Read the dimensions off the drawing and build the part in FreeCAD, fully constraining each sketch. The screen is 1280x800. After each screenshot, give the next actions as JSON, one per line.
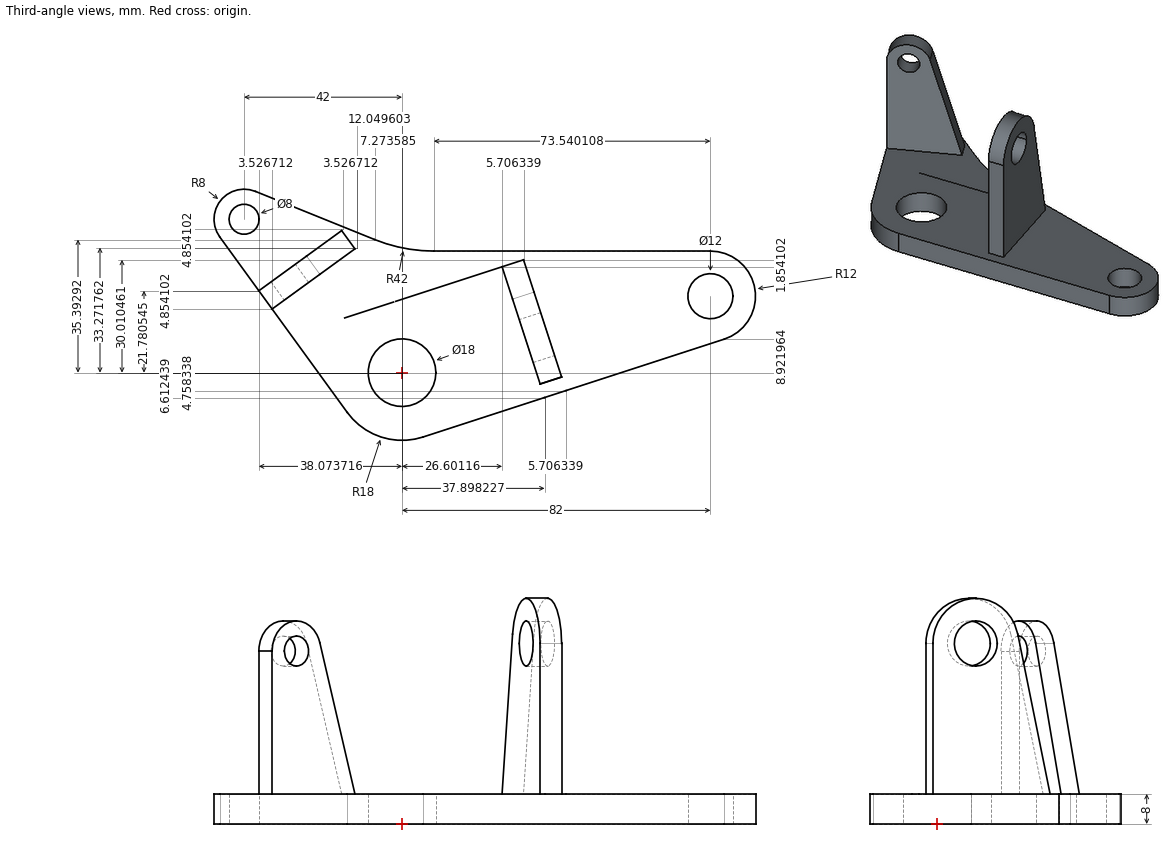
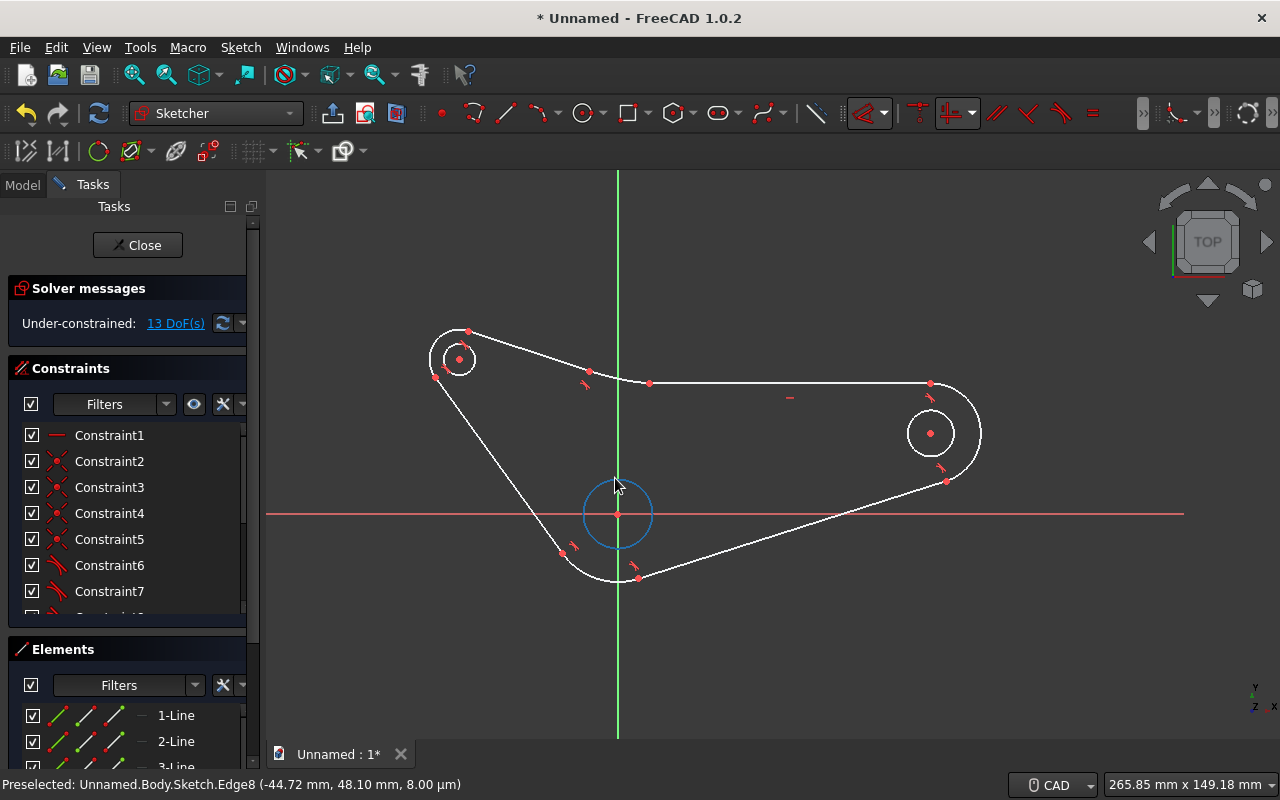
{"action": "left_click", "coordinate": [581, 571]}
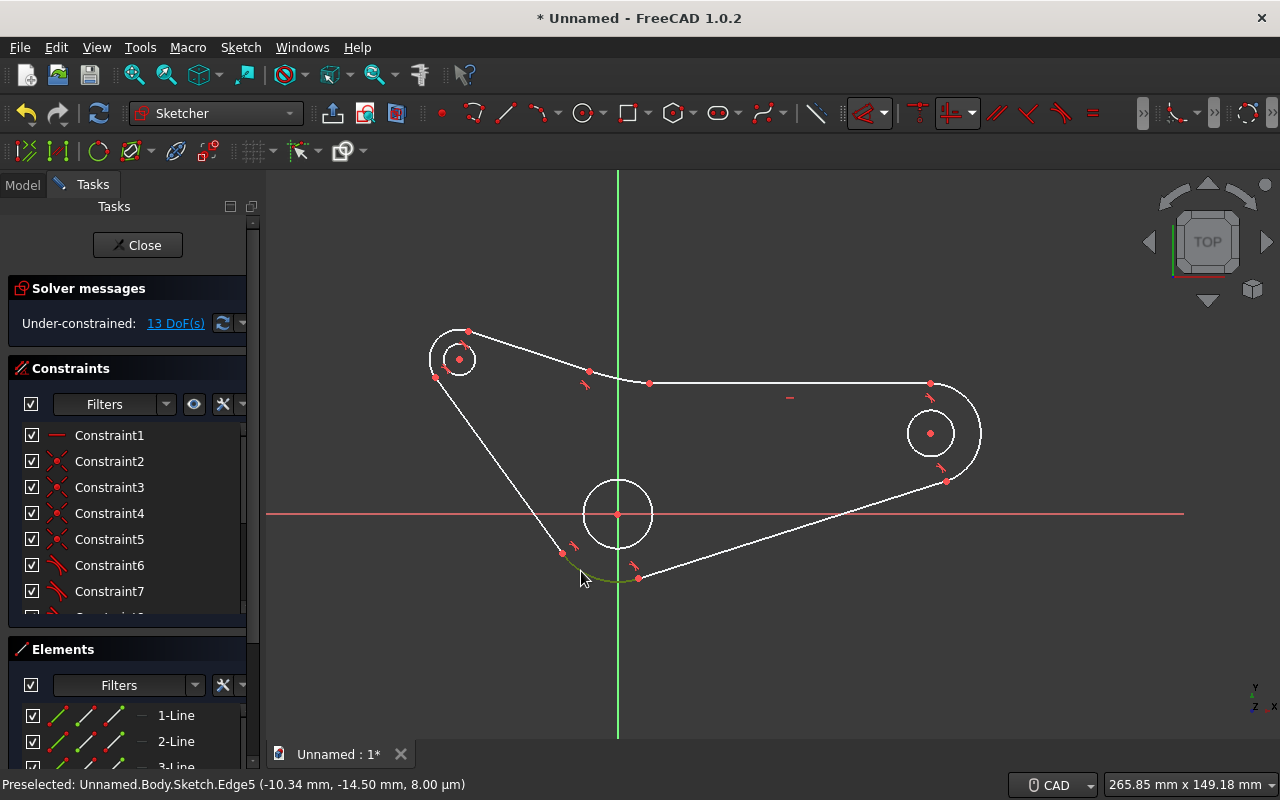
{"action": "key", "text": "k r"}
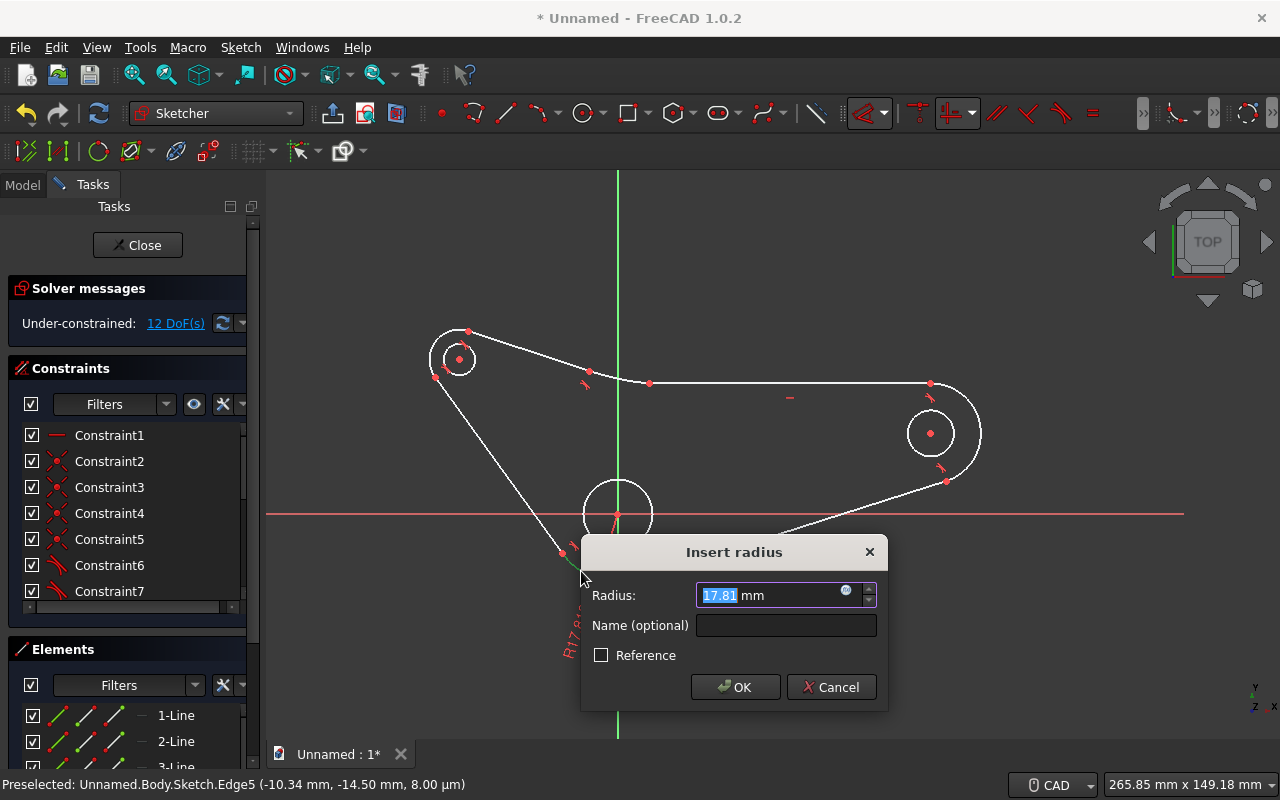
{"action": "type", "text": "18"}
{"action": "key", "text": "Return"}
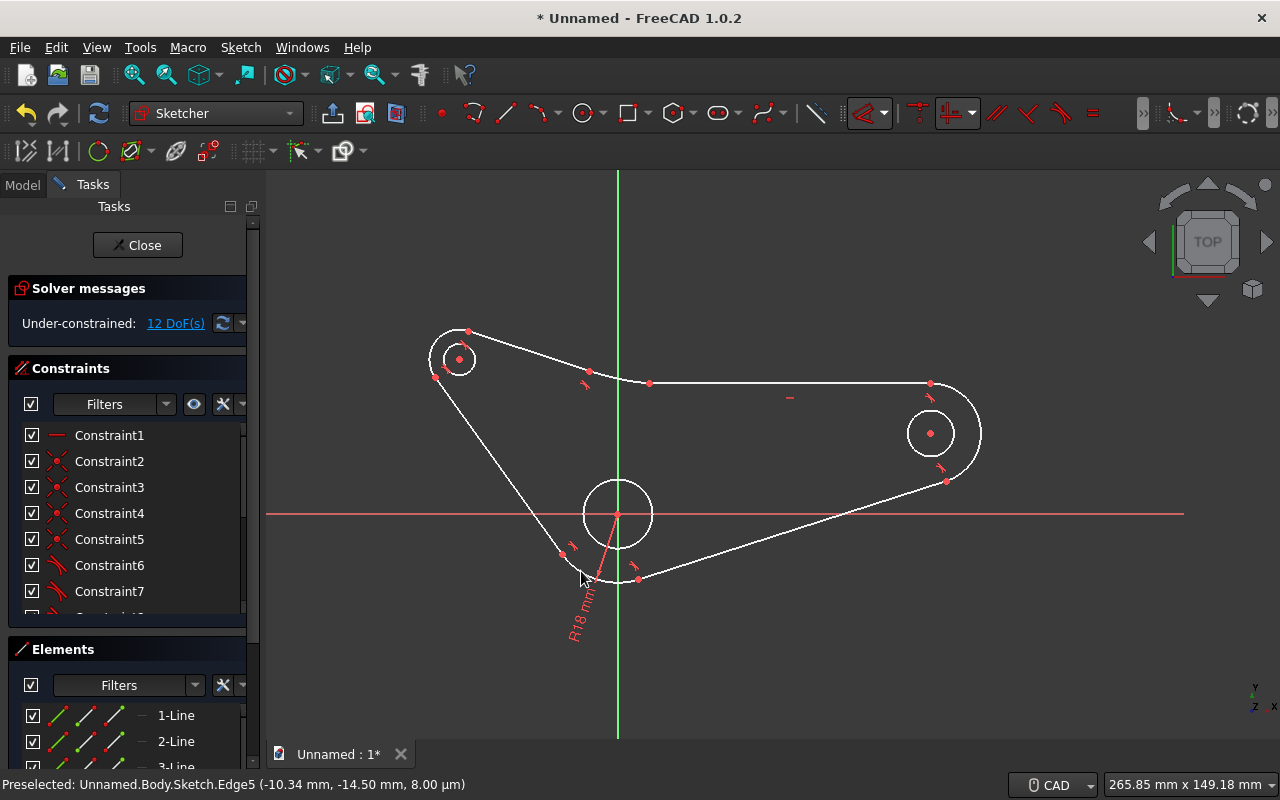
{"action": "left_click", "coordinate": [977, 453]}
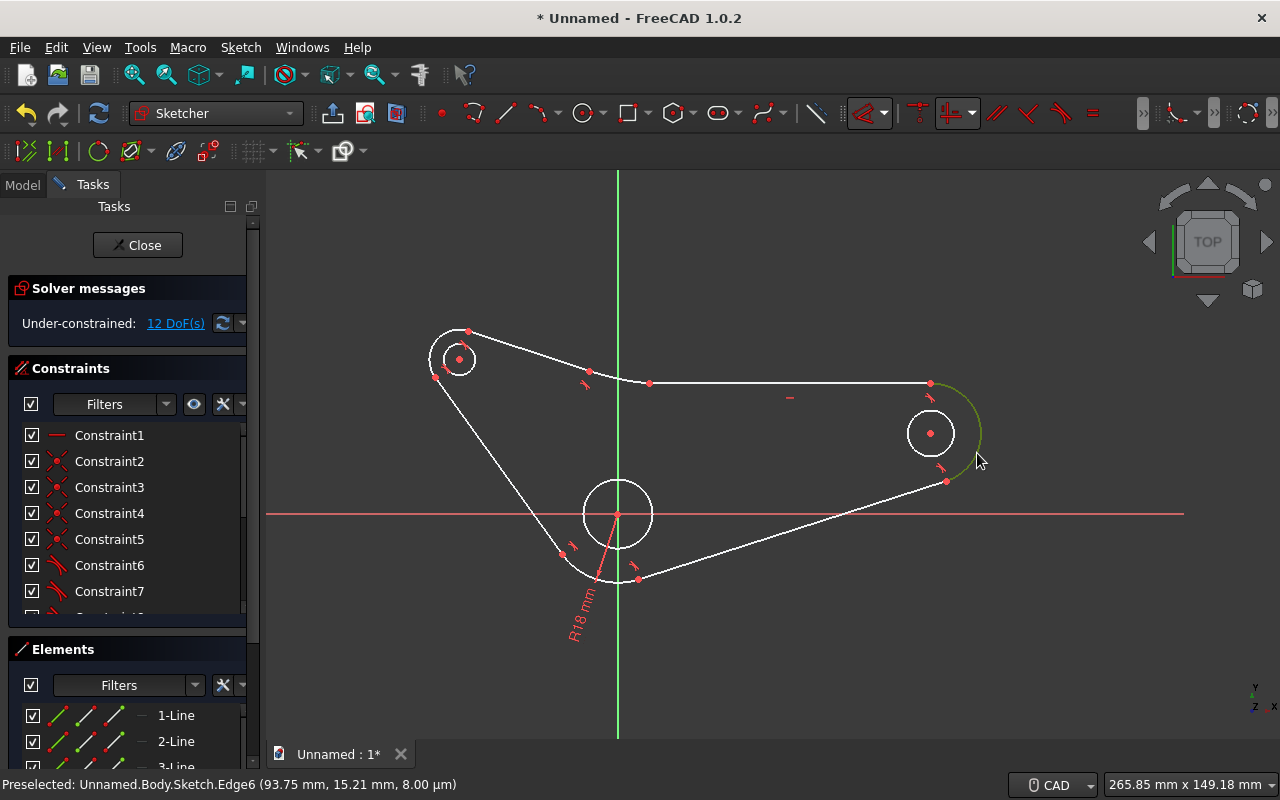
{"action": "left_click", "coordinate": [886, 114]}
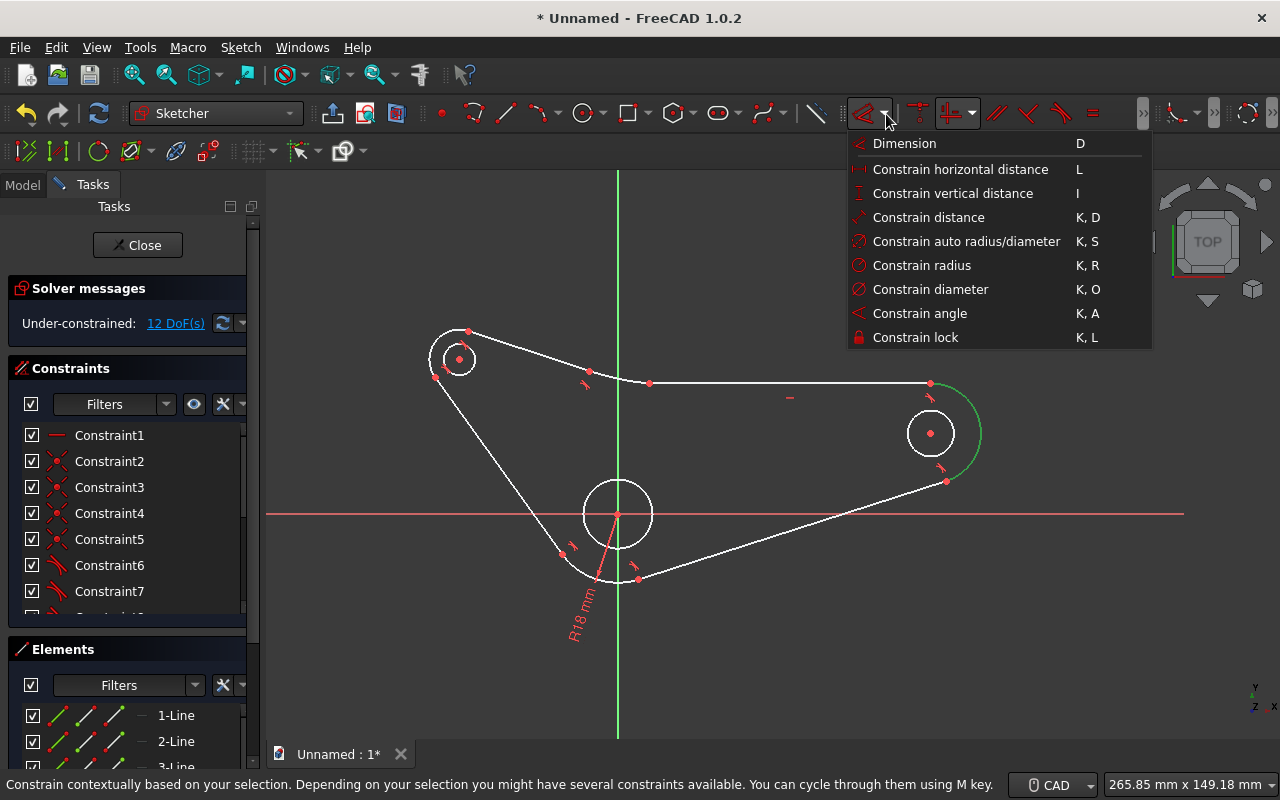
{"action": "left_click", "coordinate": [1000, 265]}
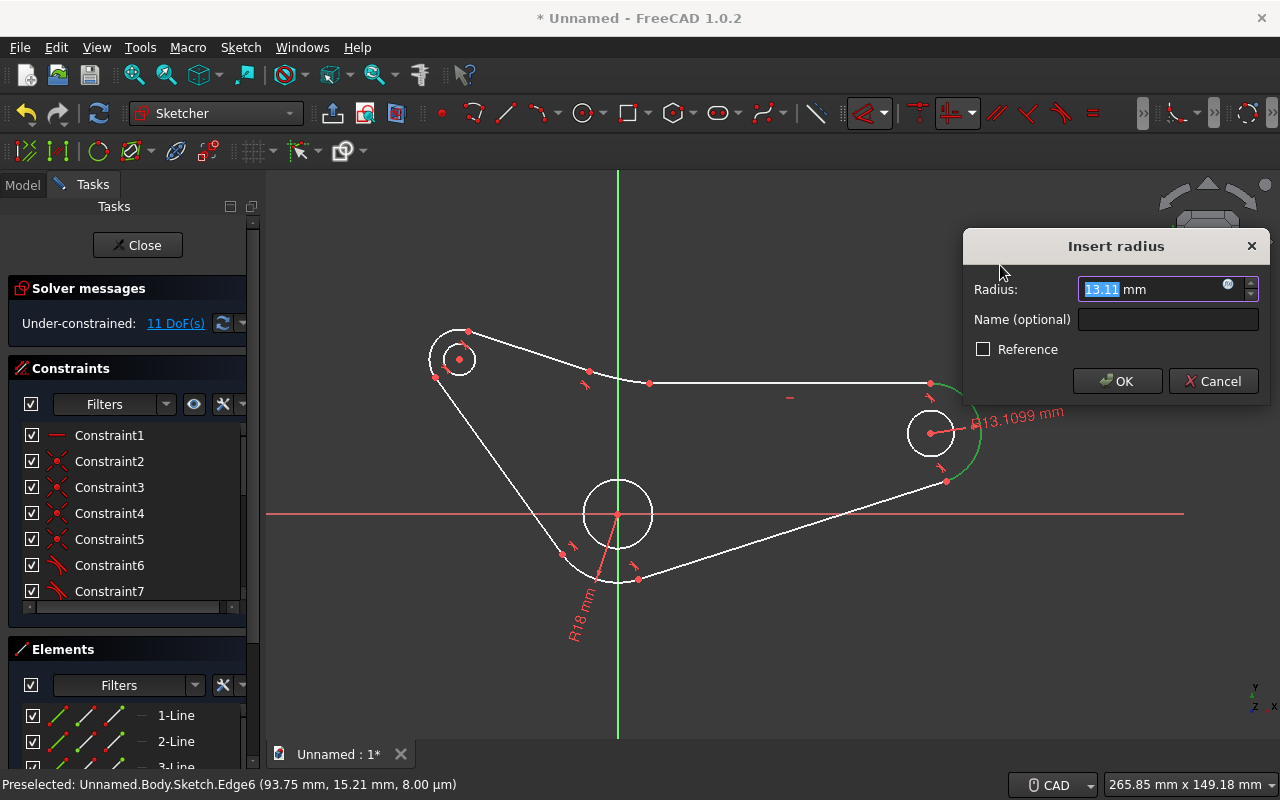
{"action": "type", "text": "12"}
{"action": "key", "text": "Return"}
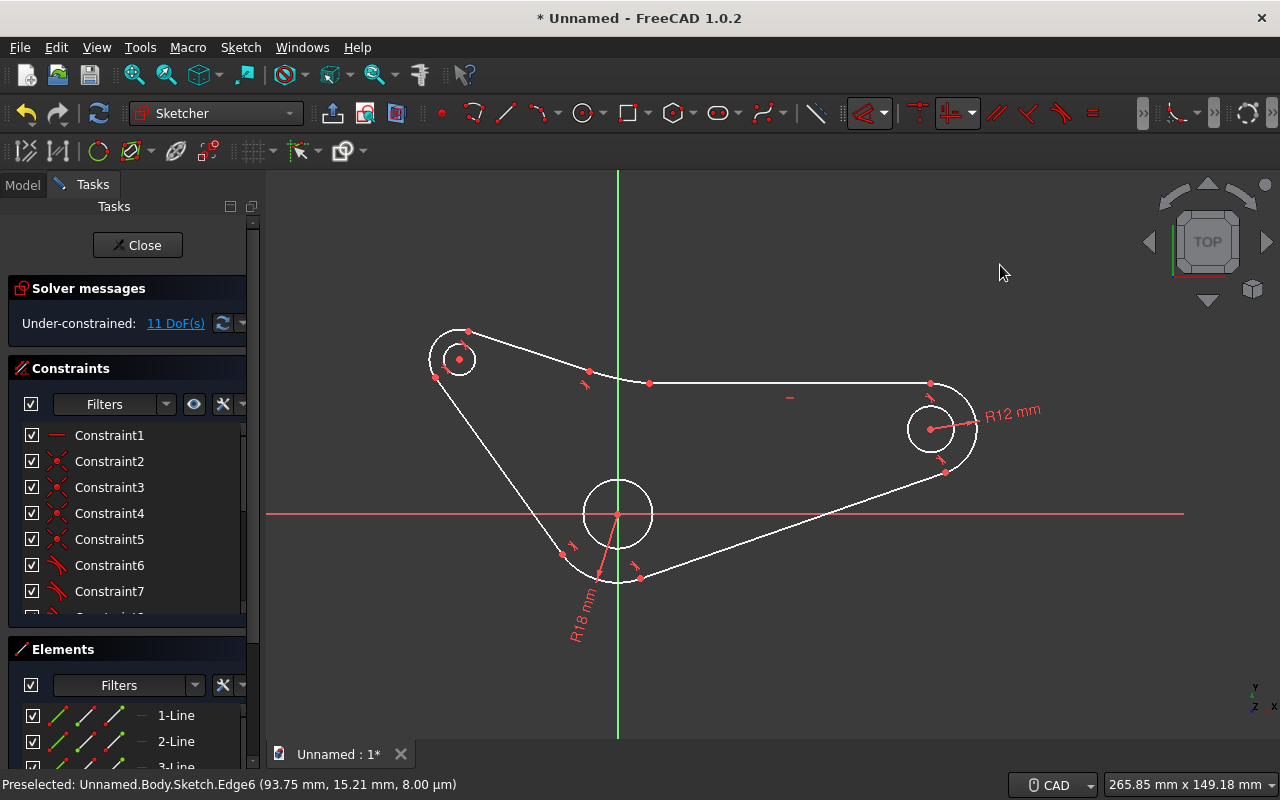
{"action": "scroll", "coordinate": [608, 376], "scroll_direction": "up", "scroll_amount": 2}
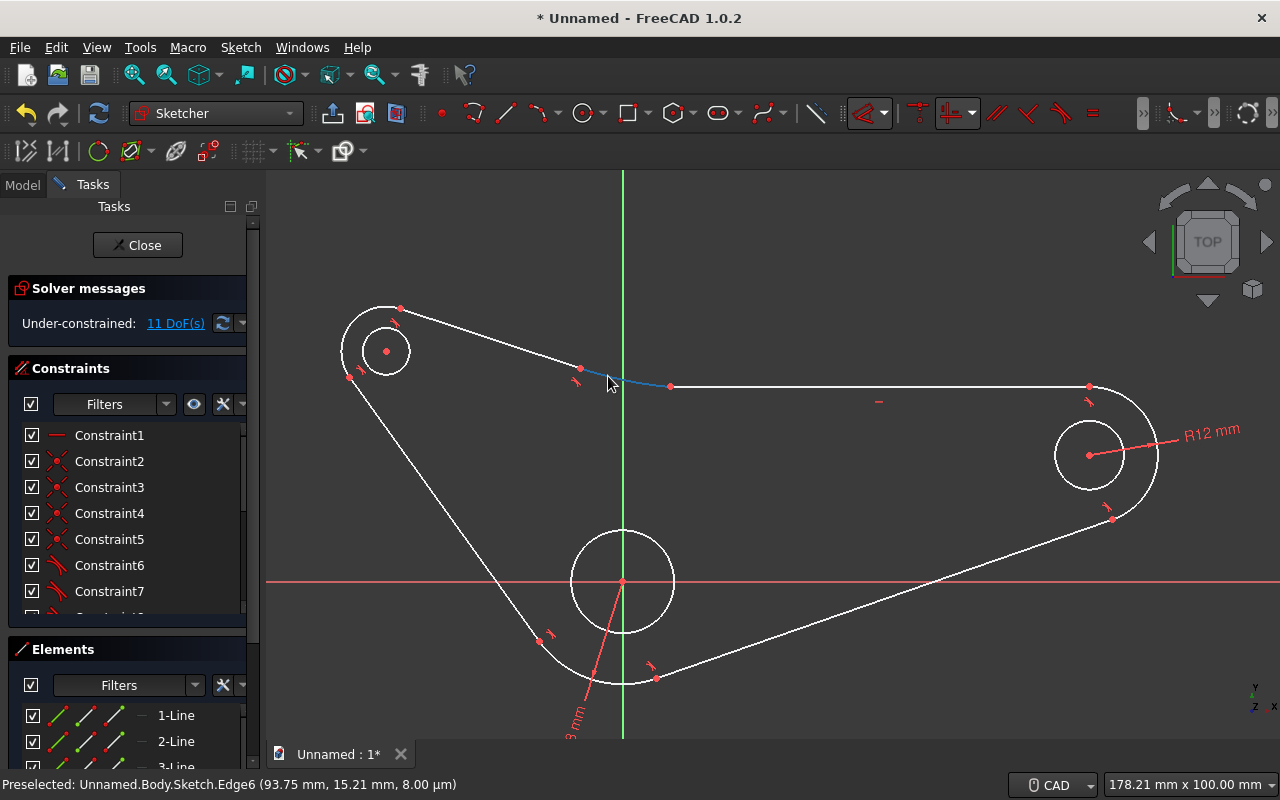
{"action": "left_click", "coordinate": [607, 376]}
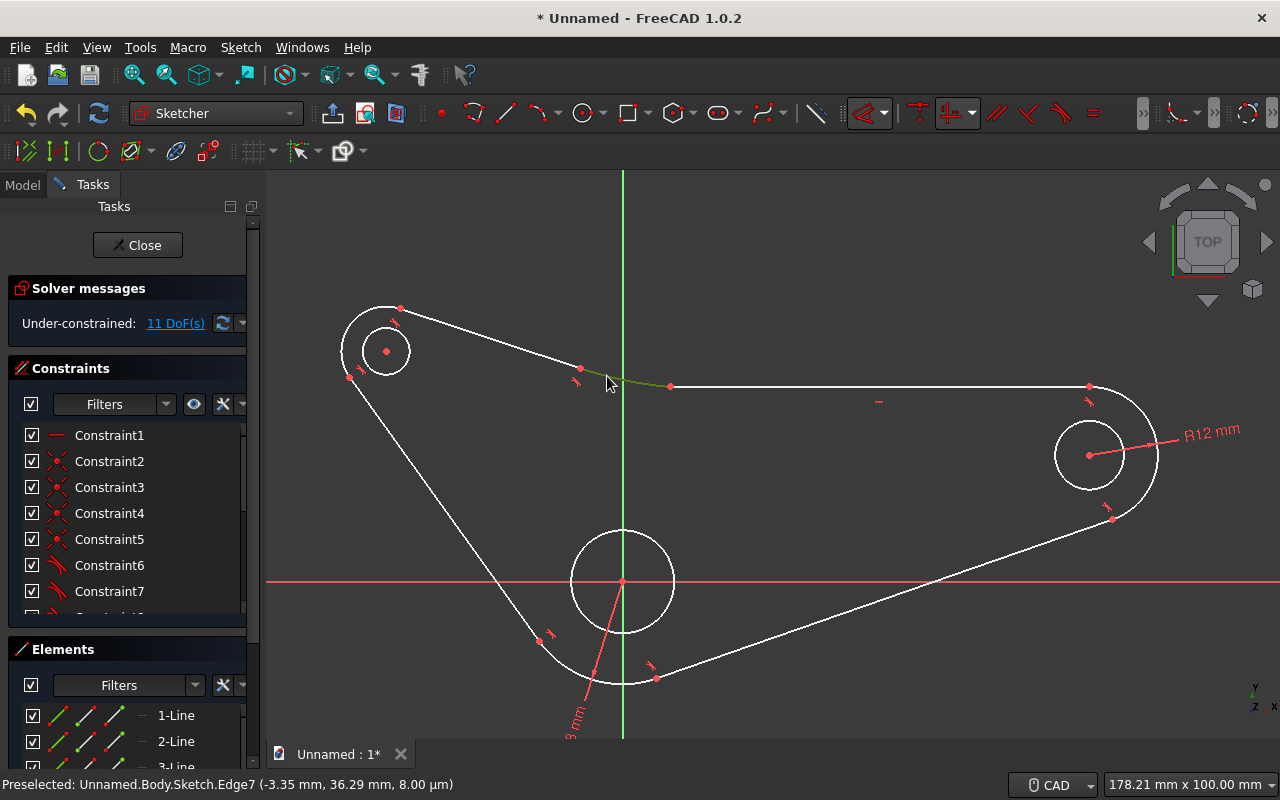
{"action": "key", "text": "k r"}